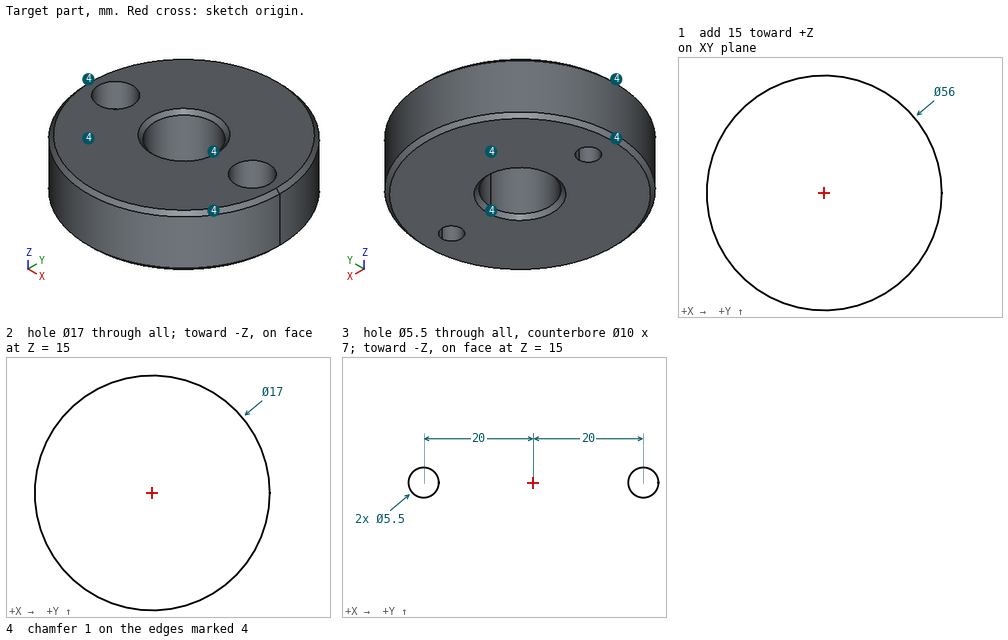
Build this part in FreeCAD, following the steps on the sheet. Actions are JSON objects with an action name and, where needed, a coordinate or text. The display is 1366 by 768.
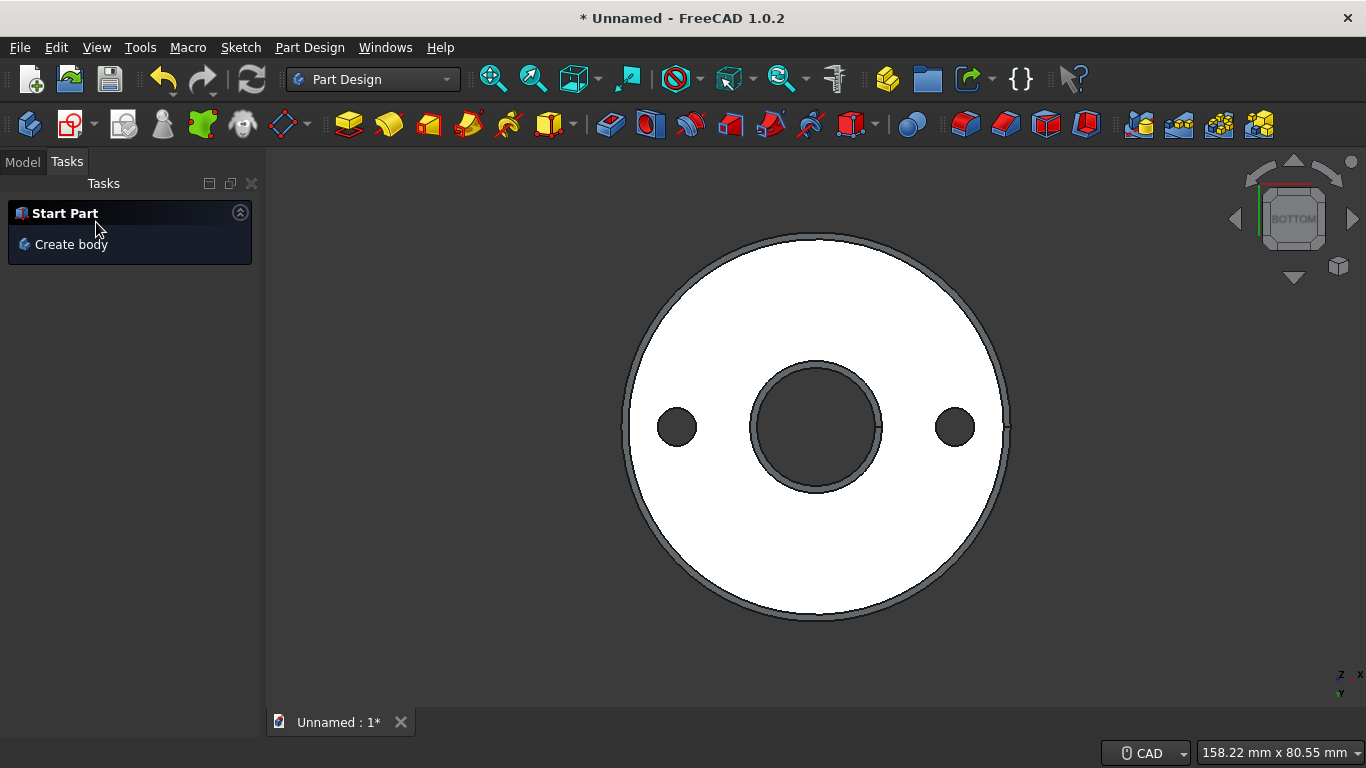
{"action": "key", "text": "0"}